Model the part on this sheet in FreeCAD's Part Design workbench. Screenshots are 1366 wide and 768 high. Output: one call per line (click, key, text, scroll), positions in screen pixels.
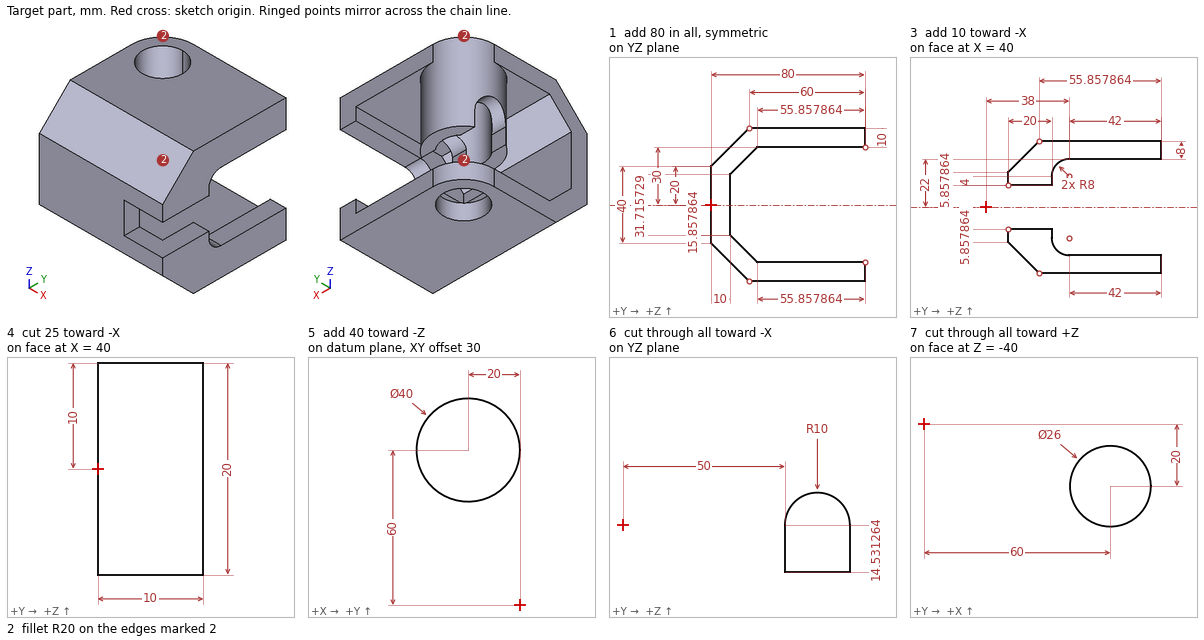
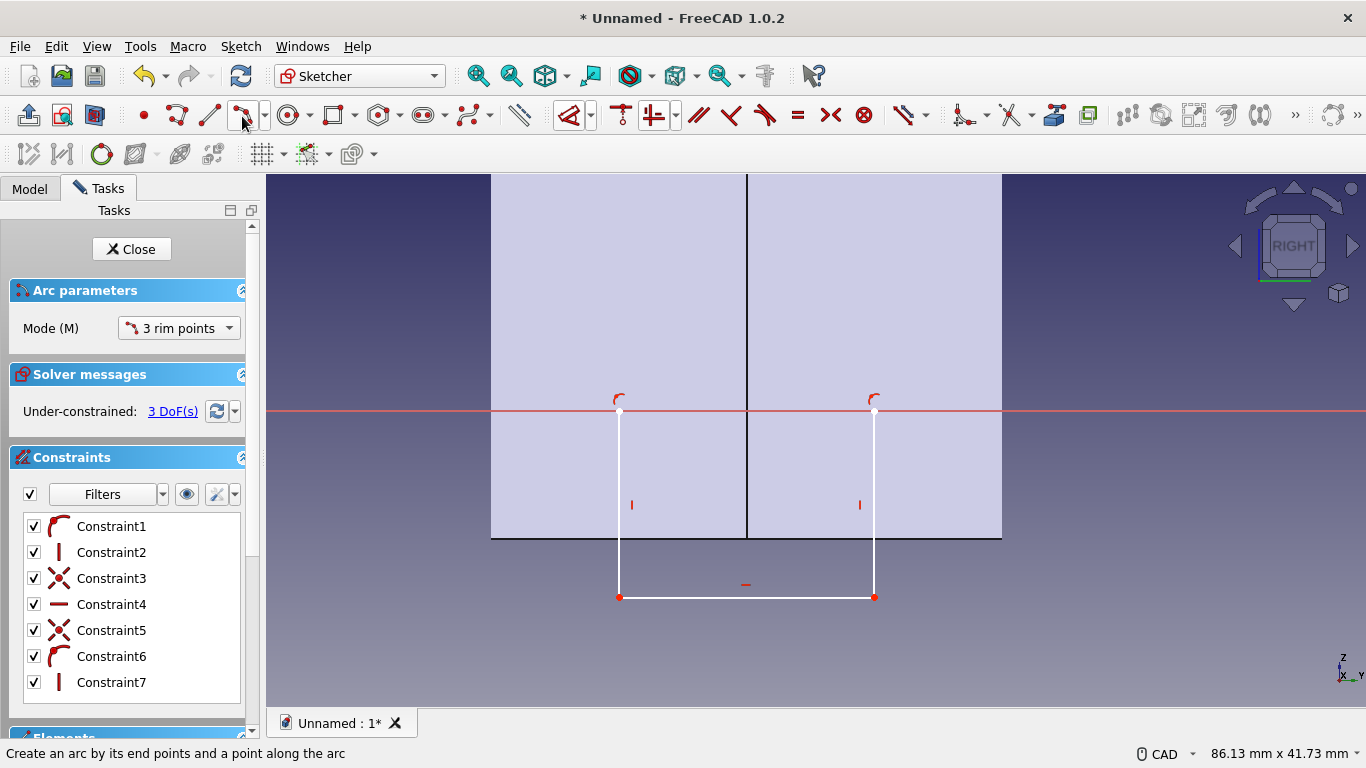
click(874, 411)
click(619, 411)
click(747, 284)
key(Escape)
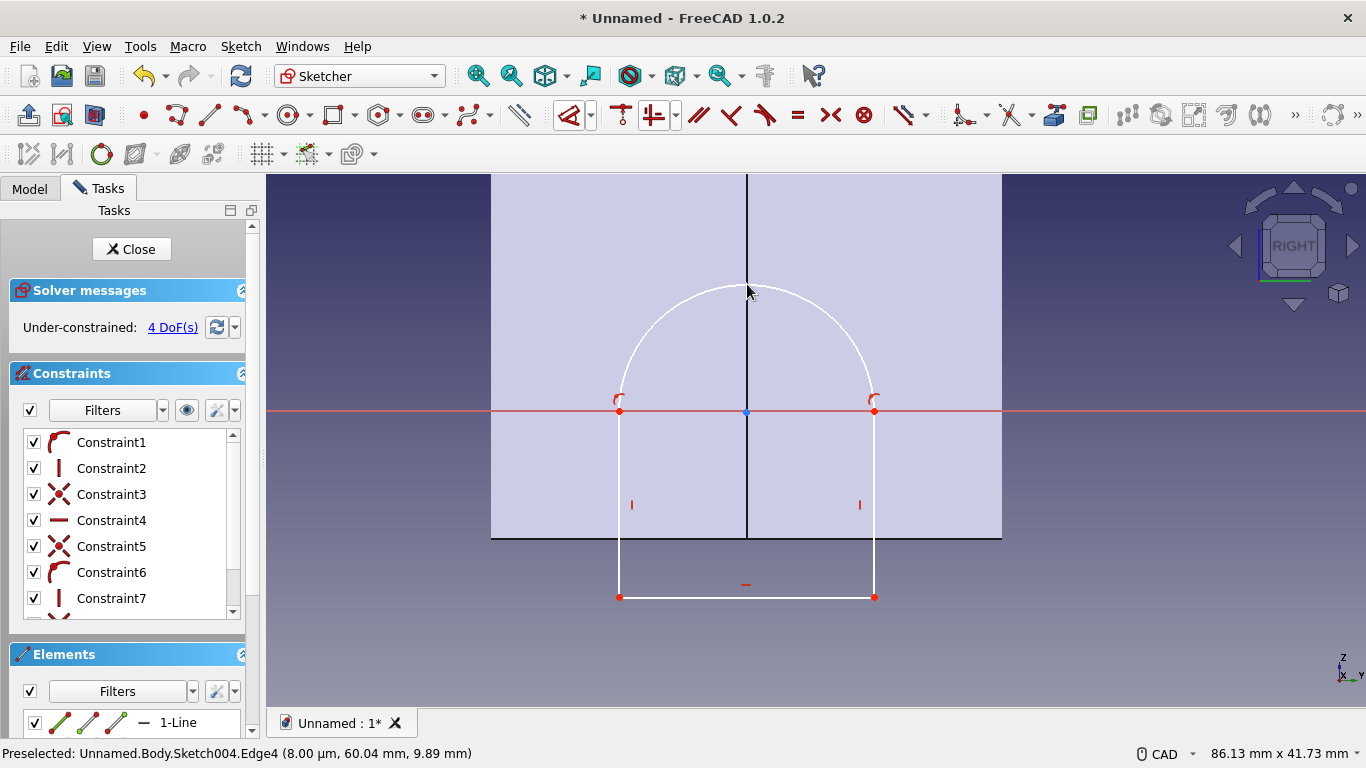
click(619, 467)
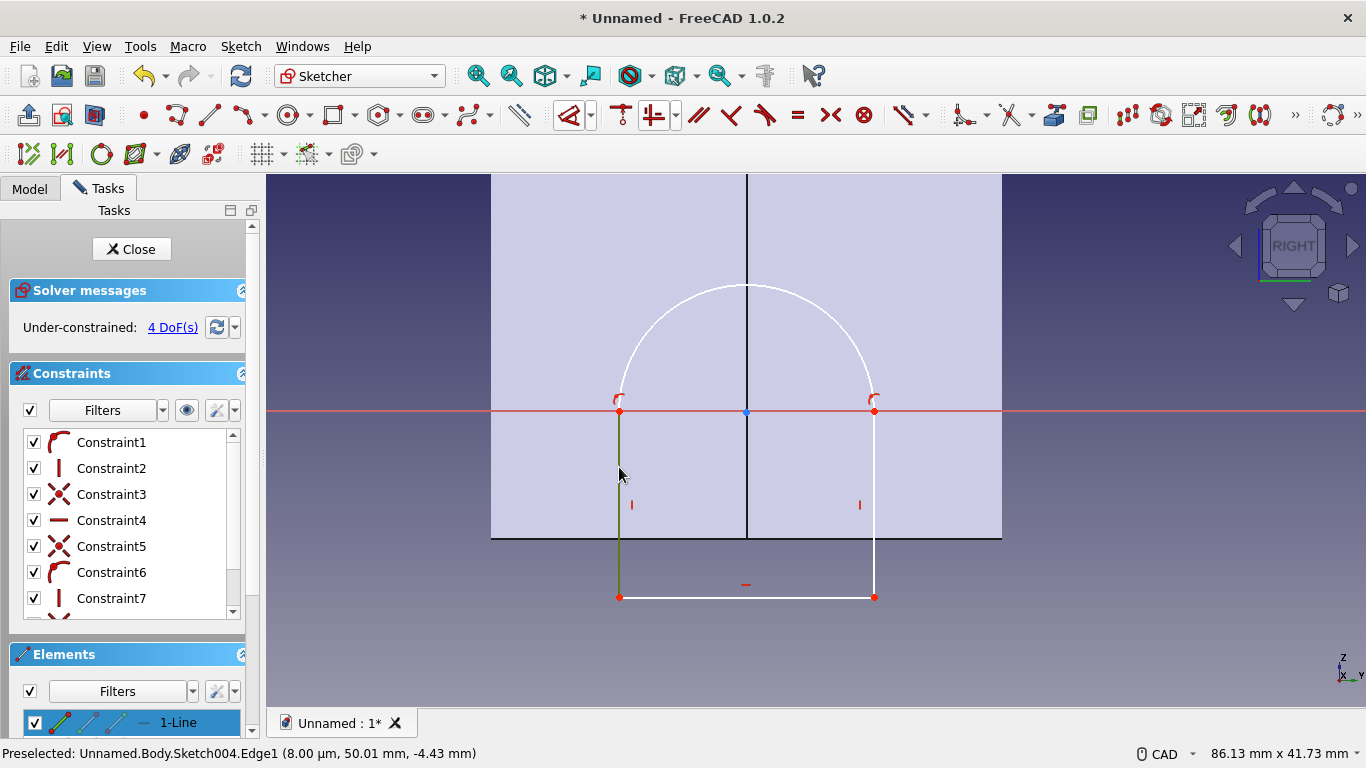
click(821, 309)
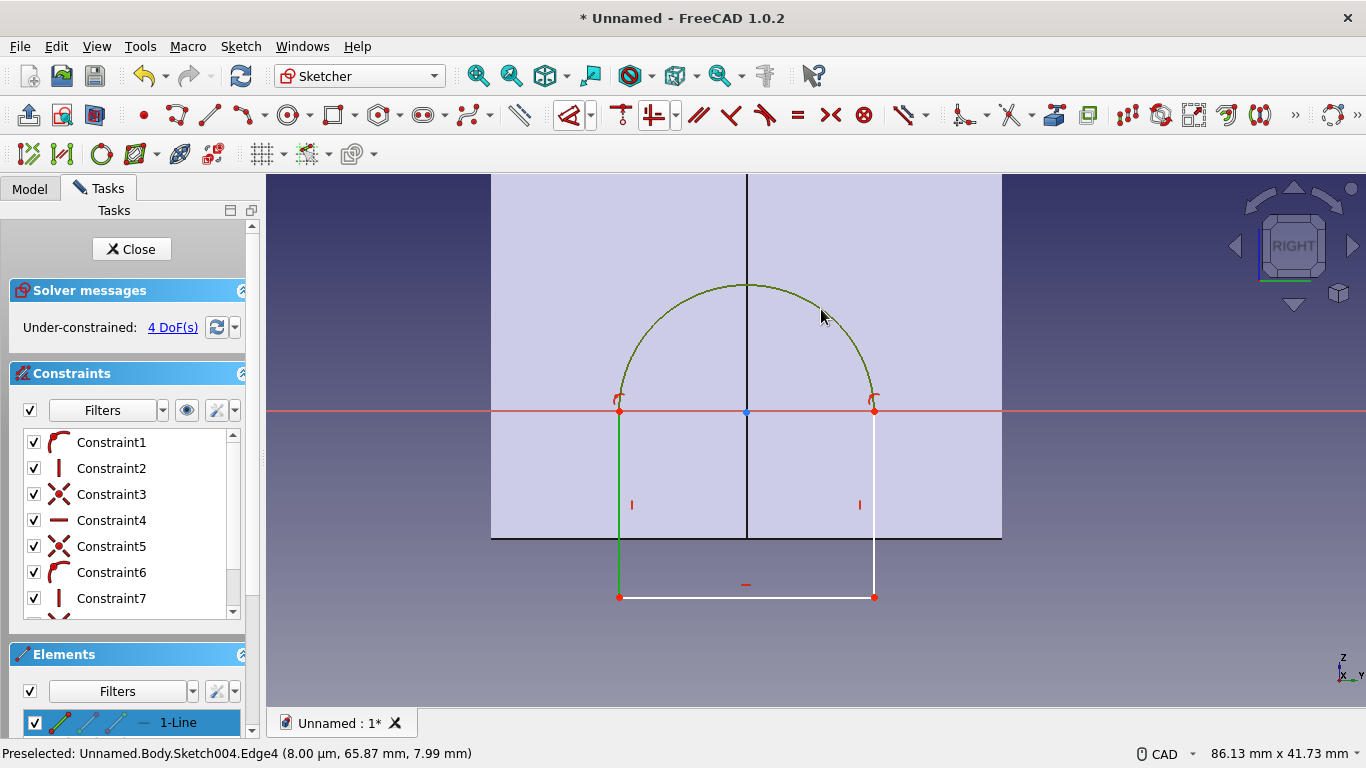
click(765, 116)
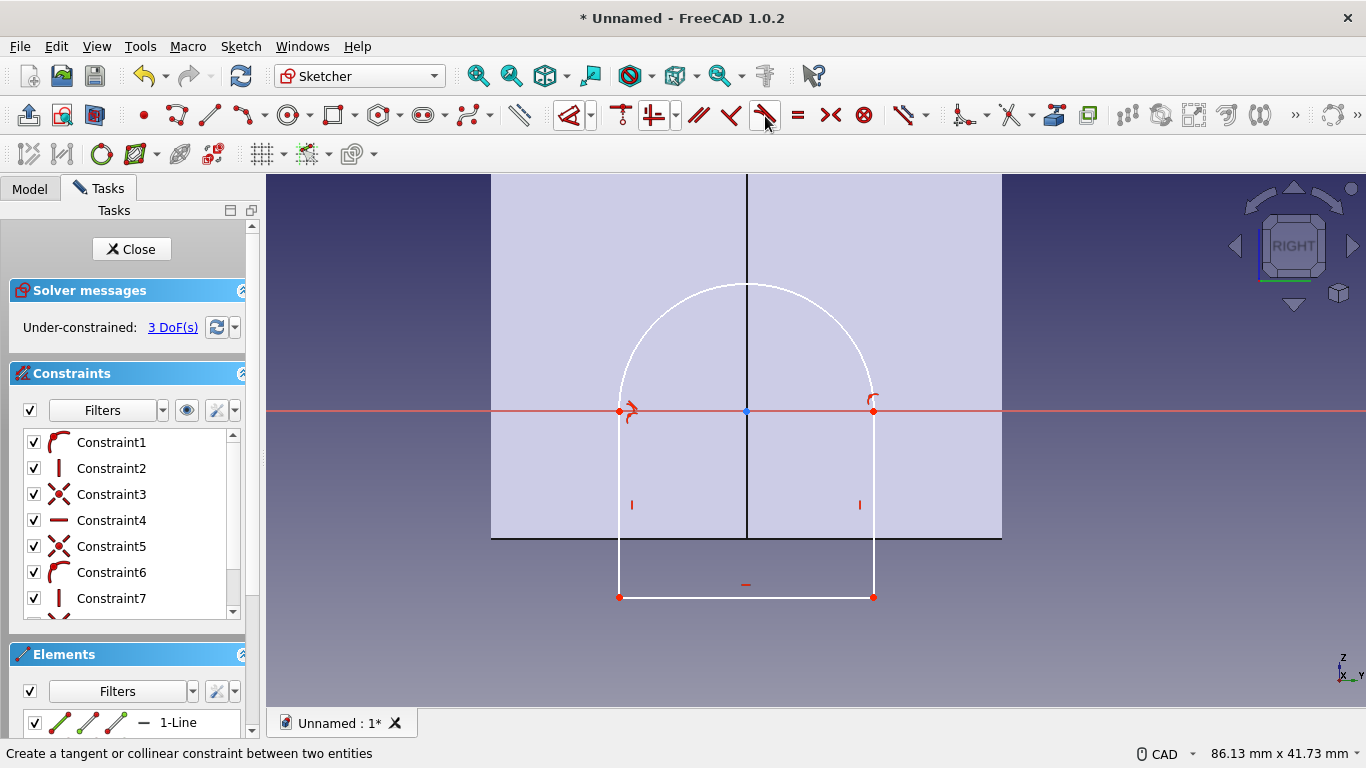
click(821, 308)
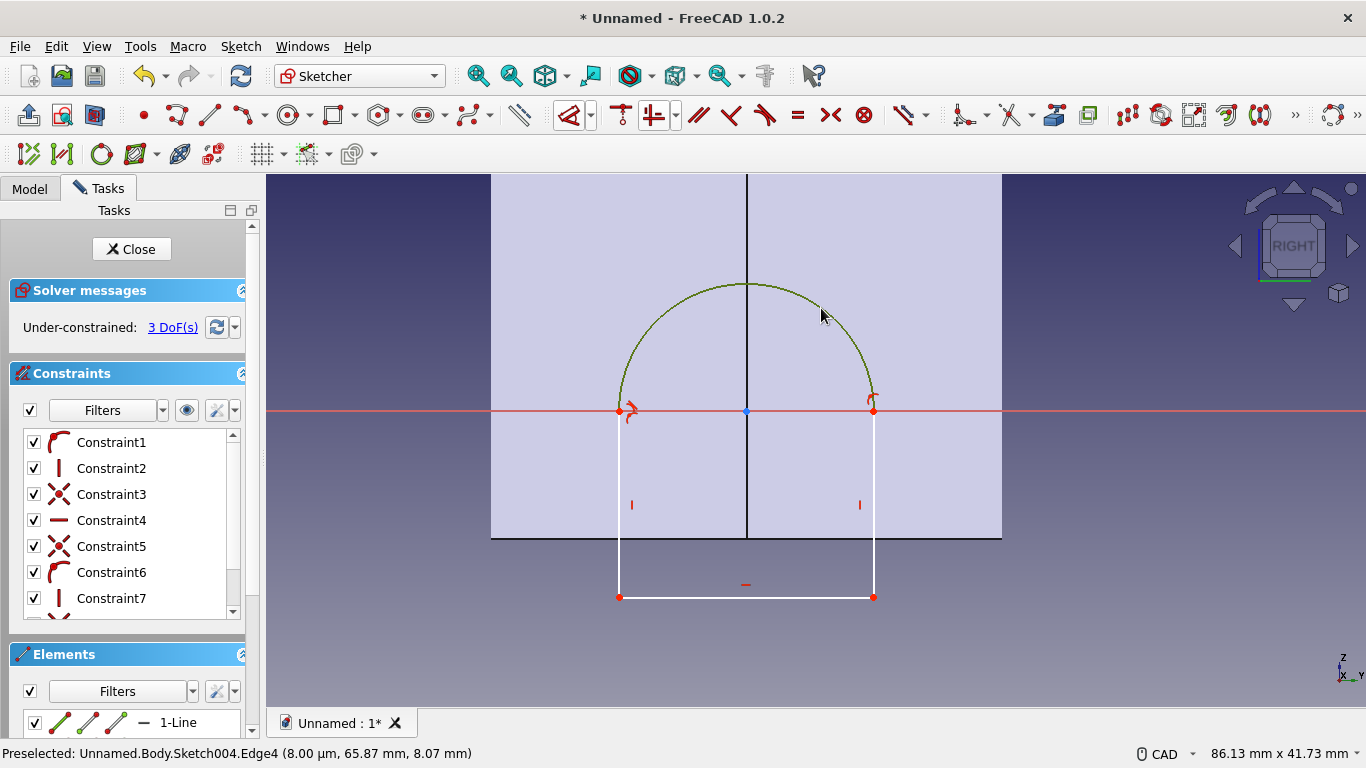
click(590, 116)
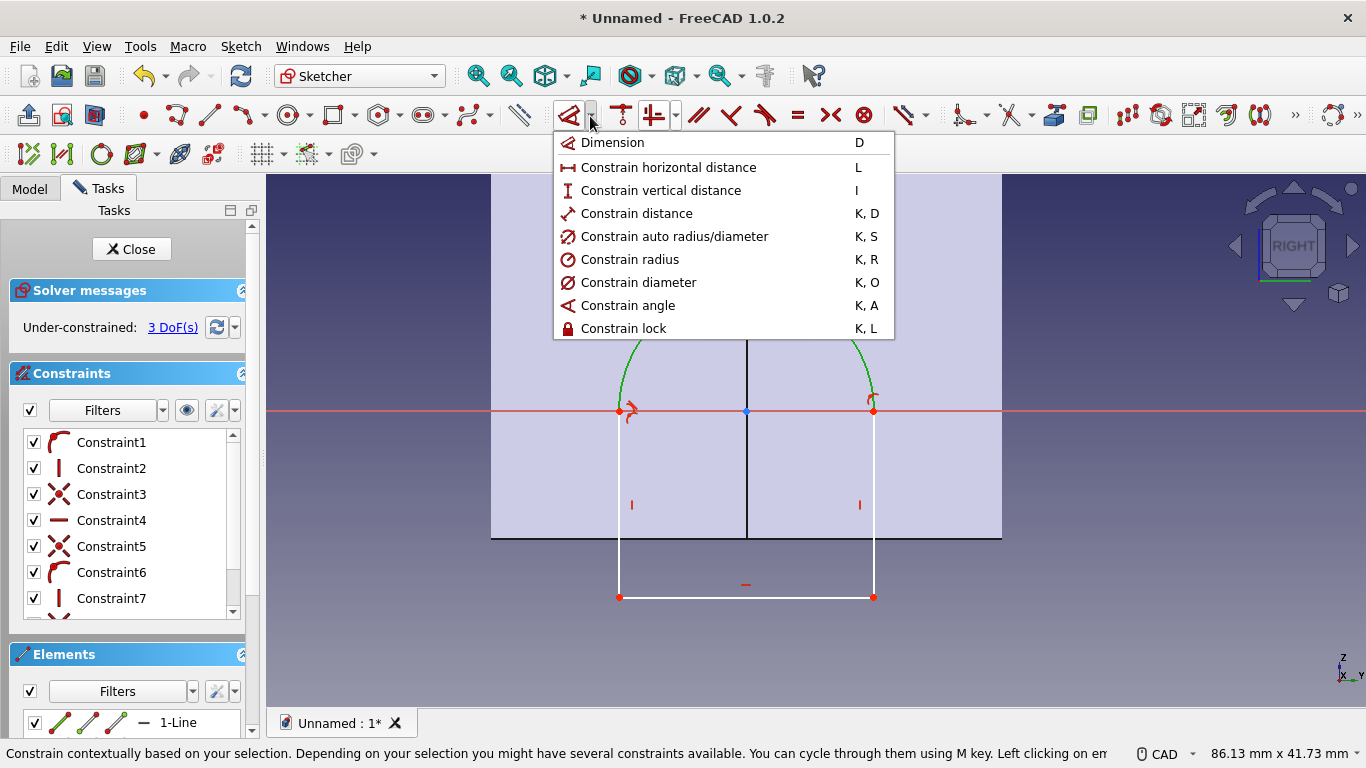
click(724, 260)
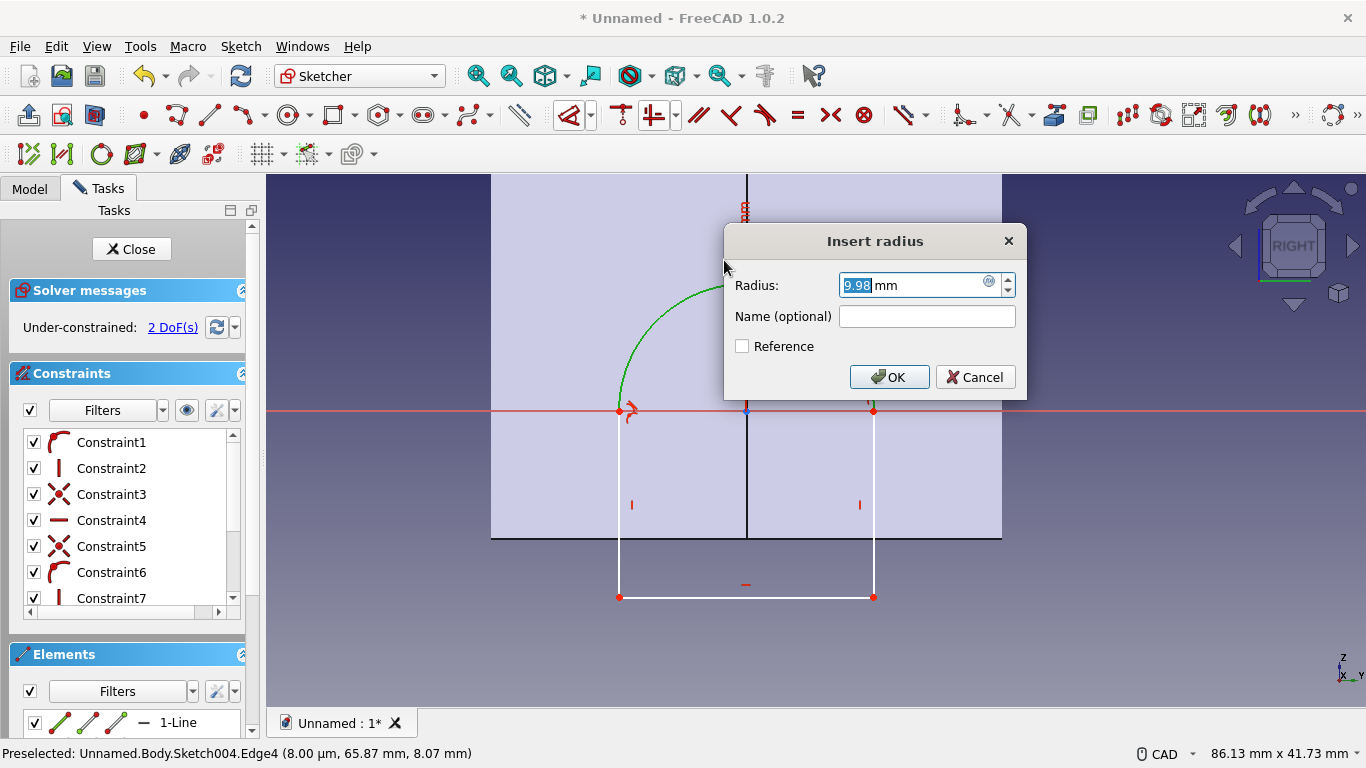
text(10)
key(Return)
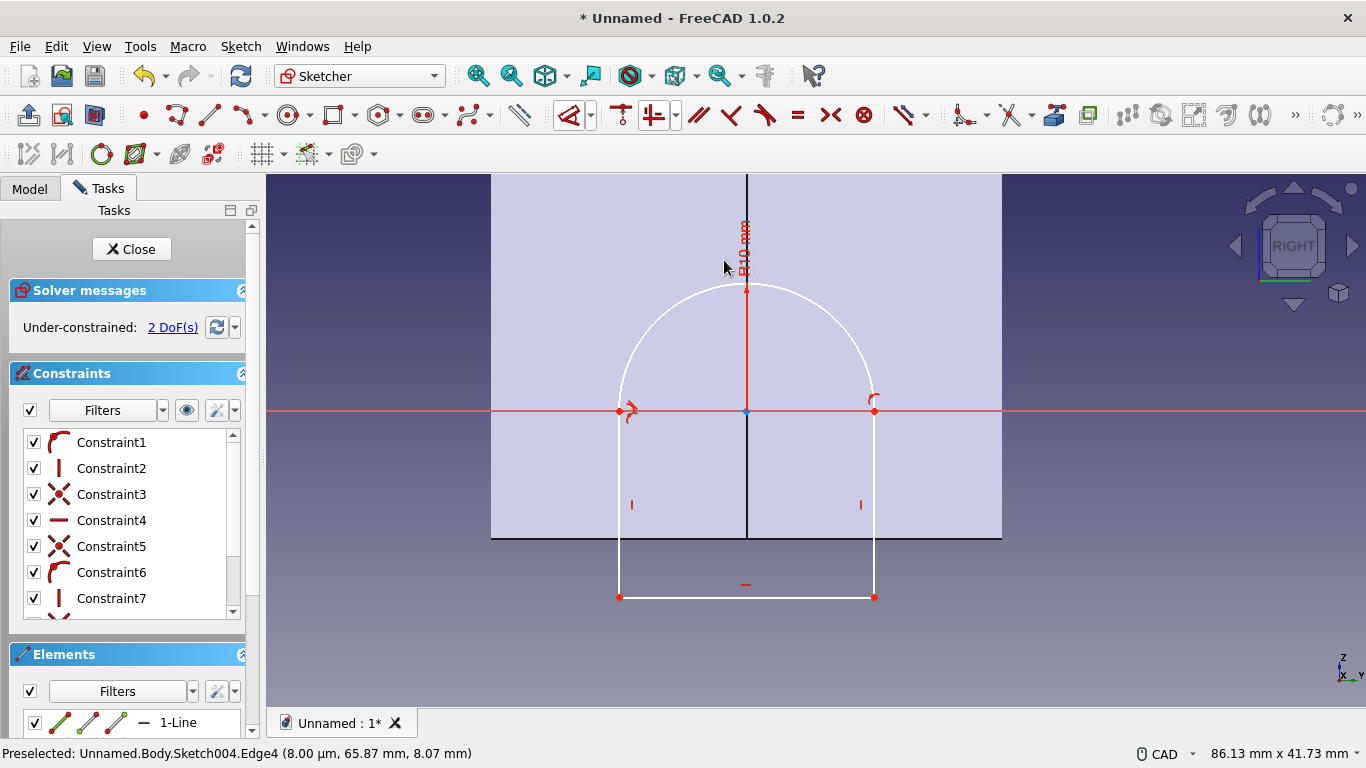
click(619, 411)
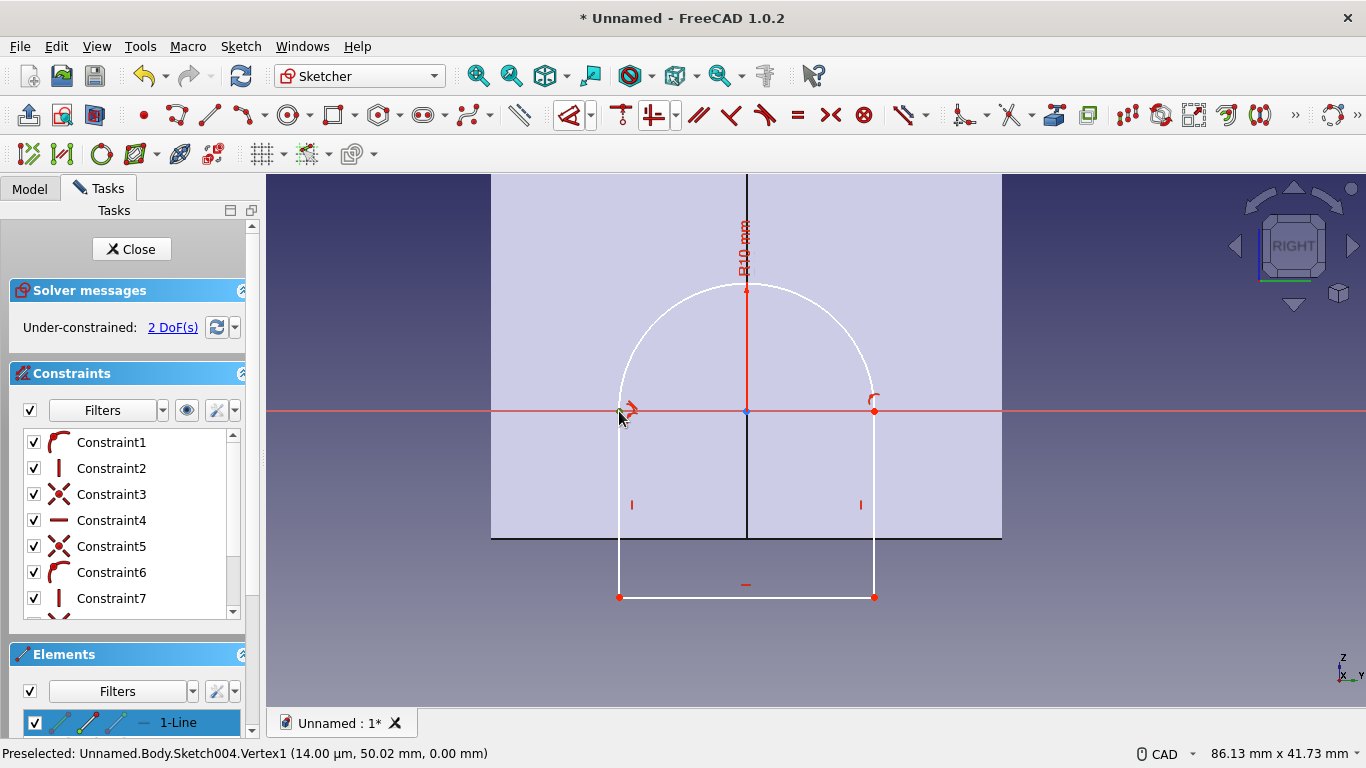
key(l)